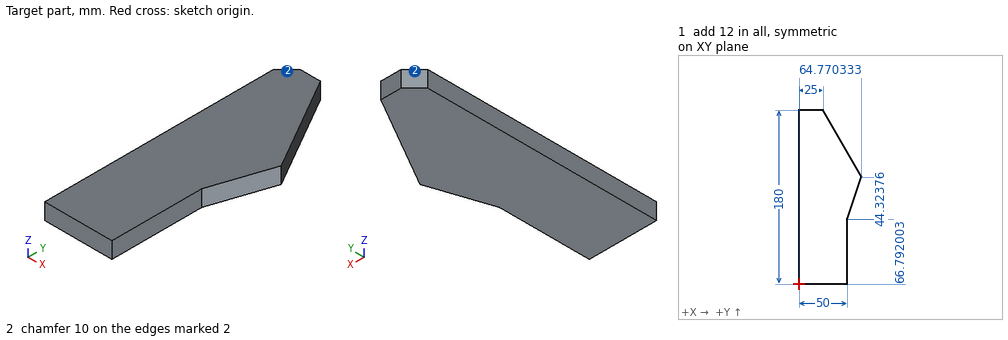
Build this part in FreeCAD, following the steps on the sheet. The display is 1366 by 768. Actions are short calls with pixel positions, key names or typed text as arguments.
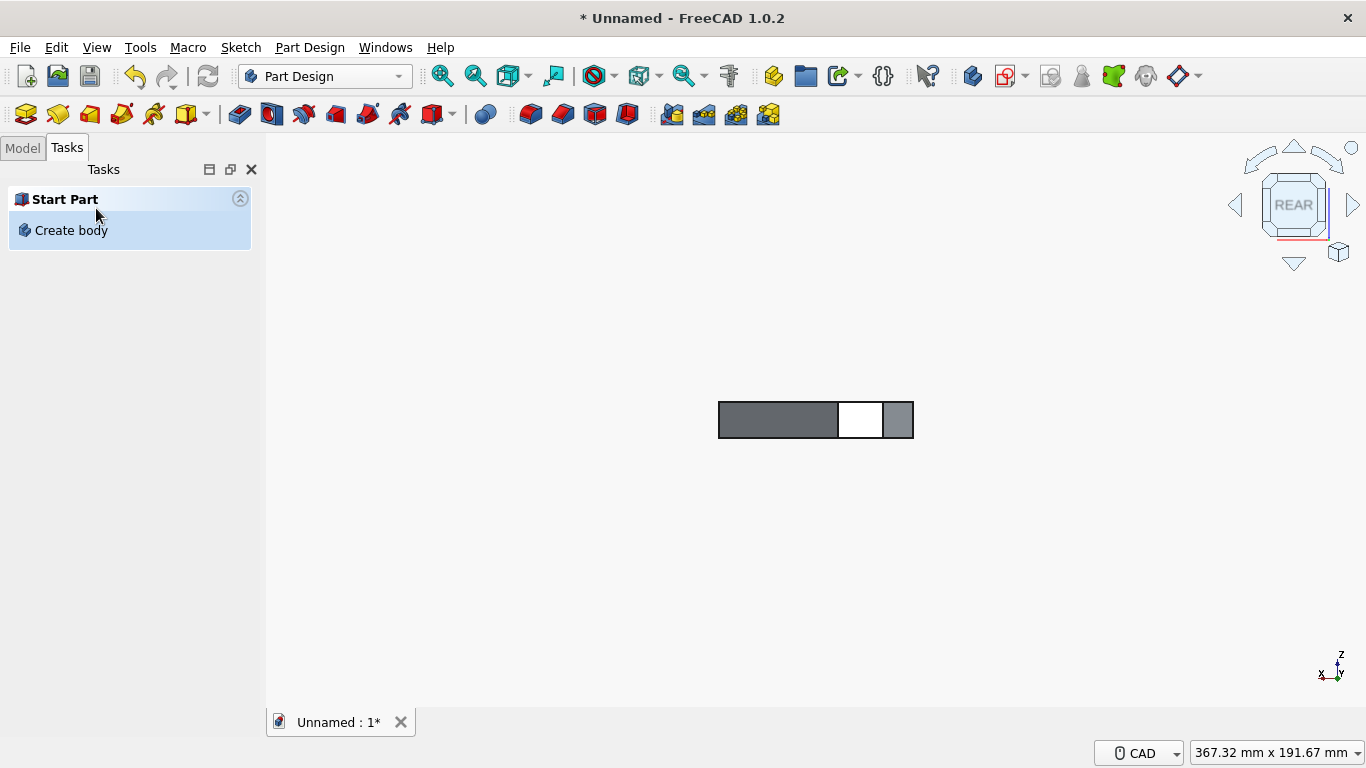
key(0)